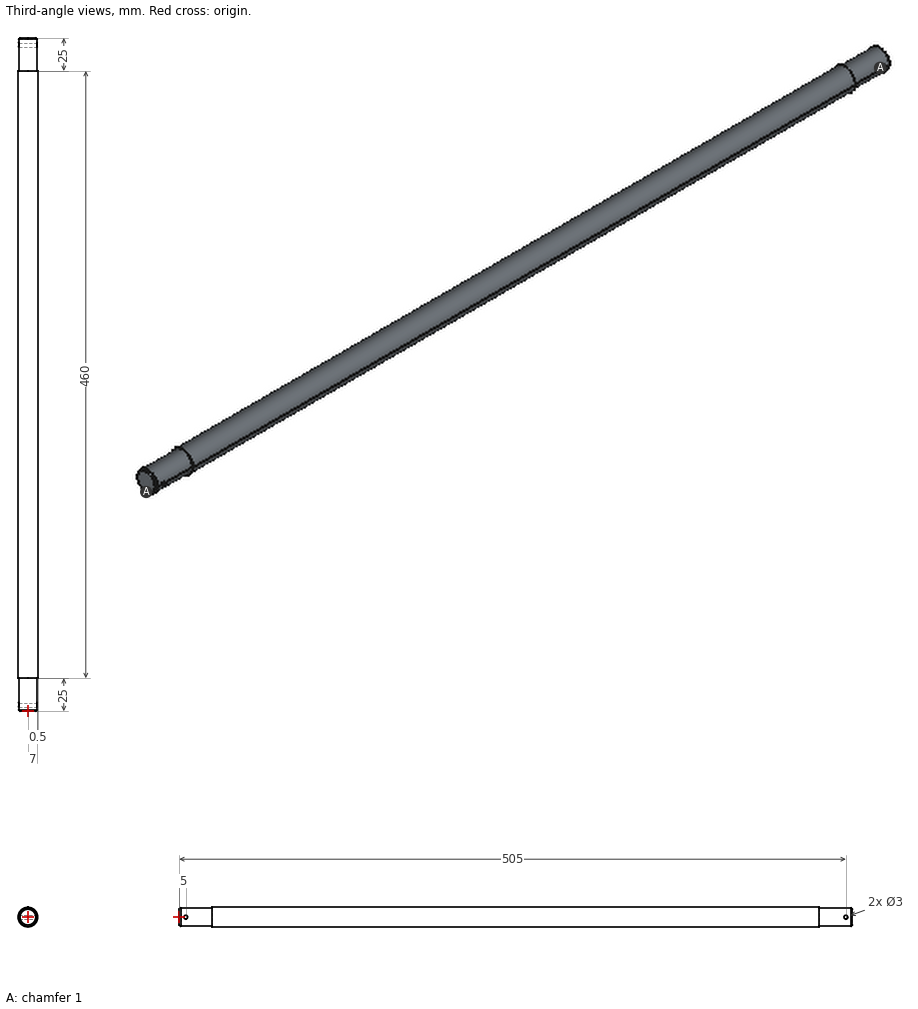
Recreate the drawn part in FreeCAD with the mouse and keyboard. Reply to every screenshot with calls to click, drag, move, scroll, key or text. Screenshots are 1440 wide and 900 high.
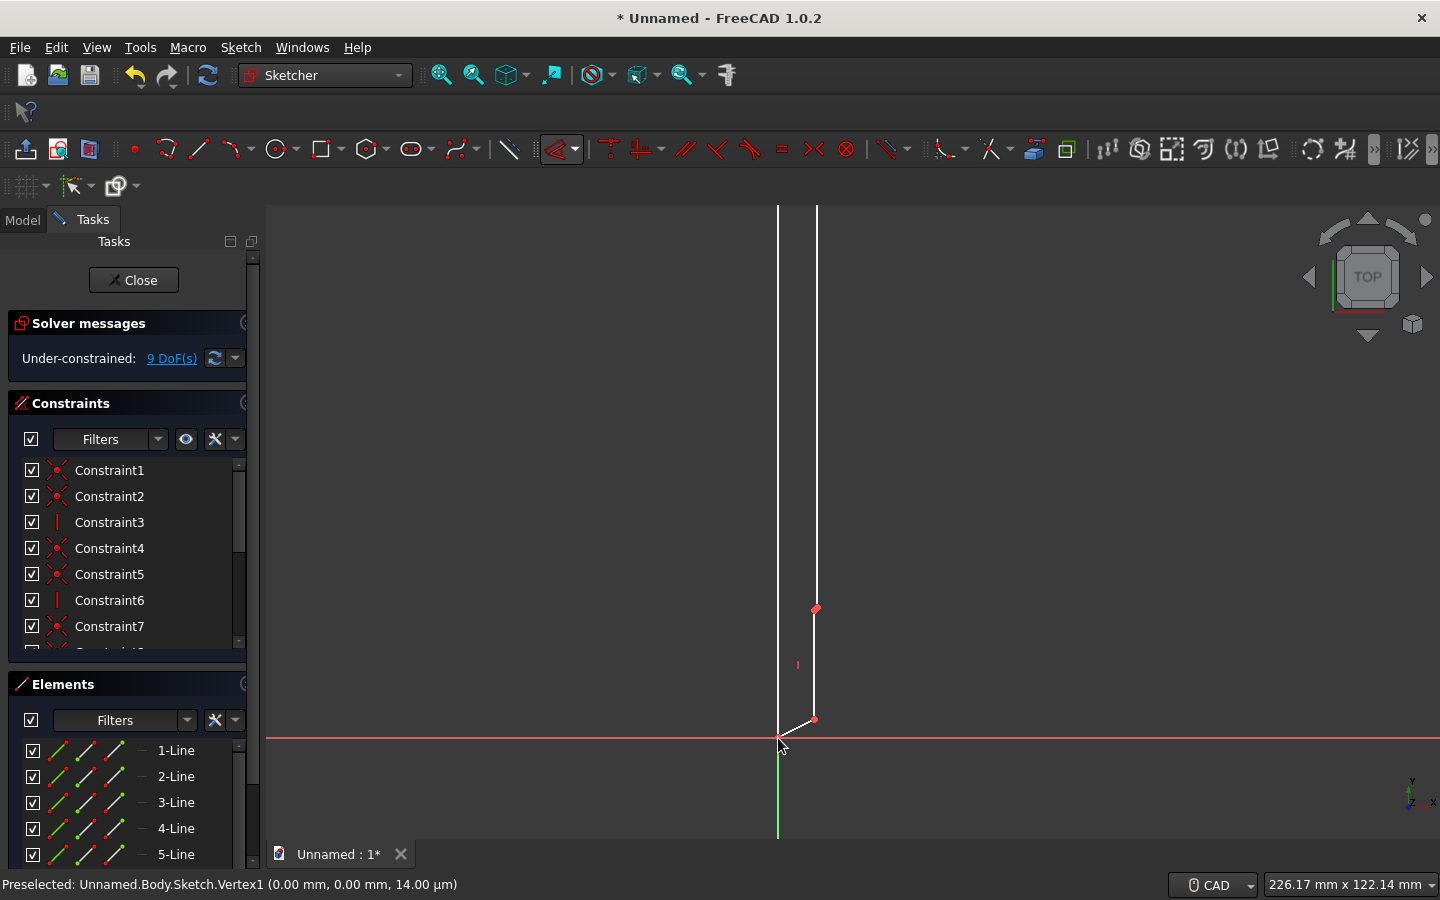
click(804, 725)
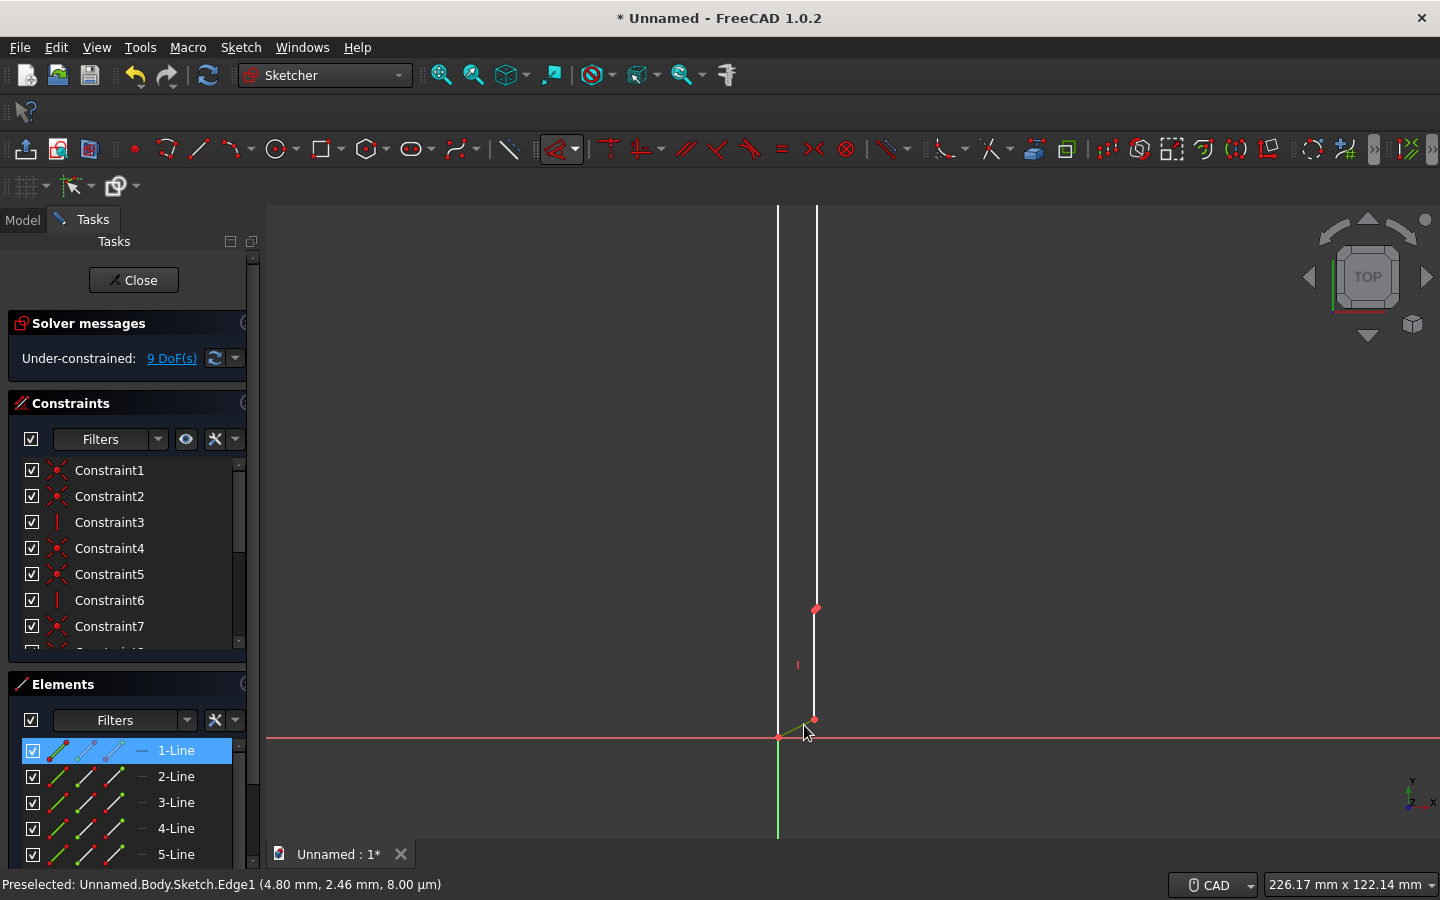
click(664, 150)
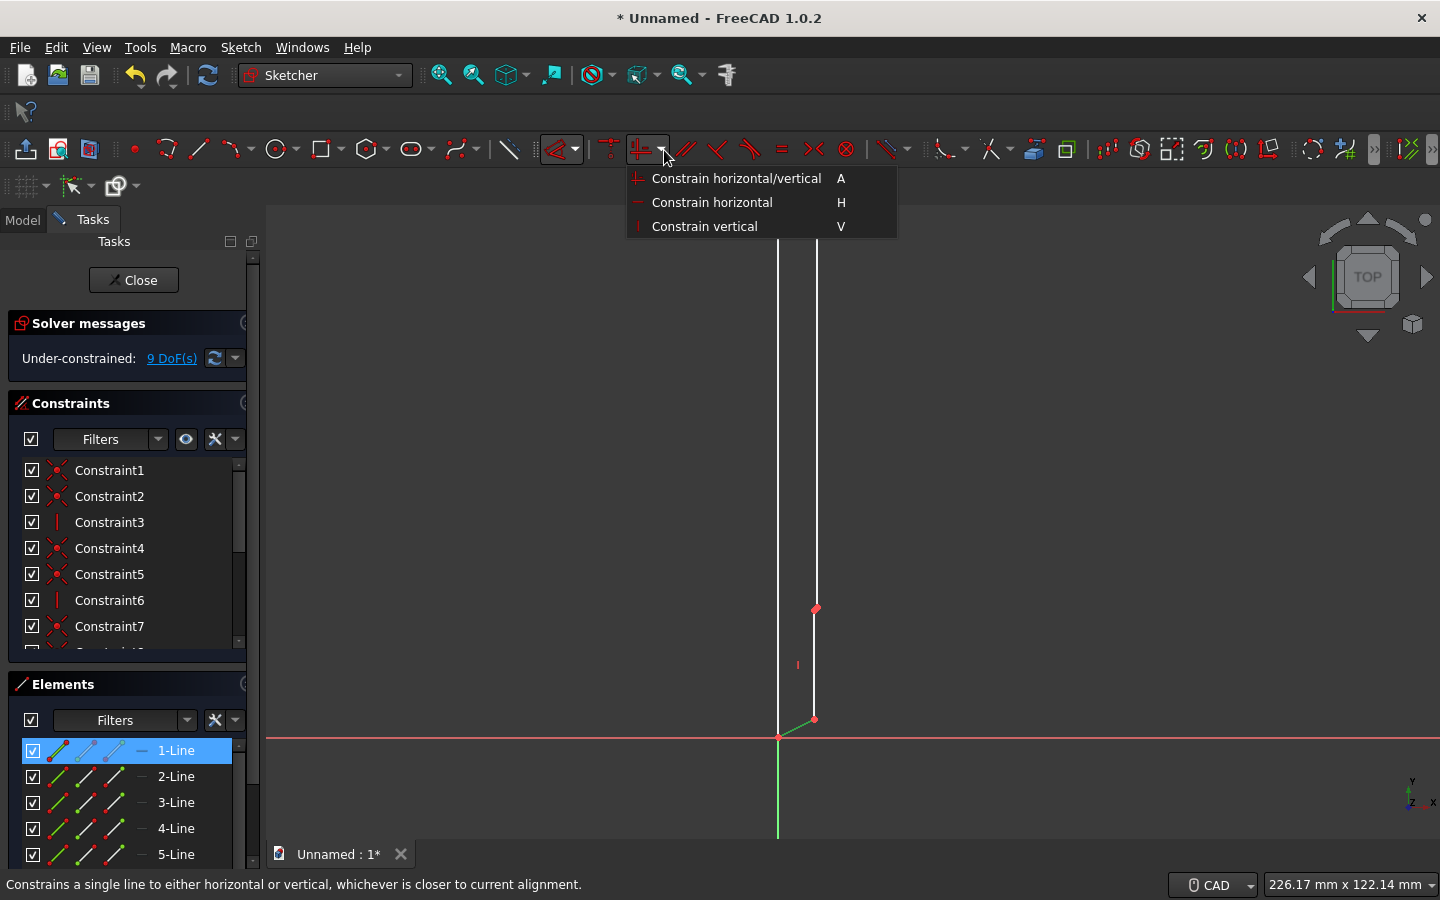
click(762, 202)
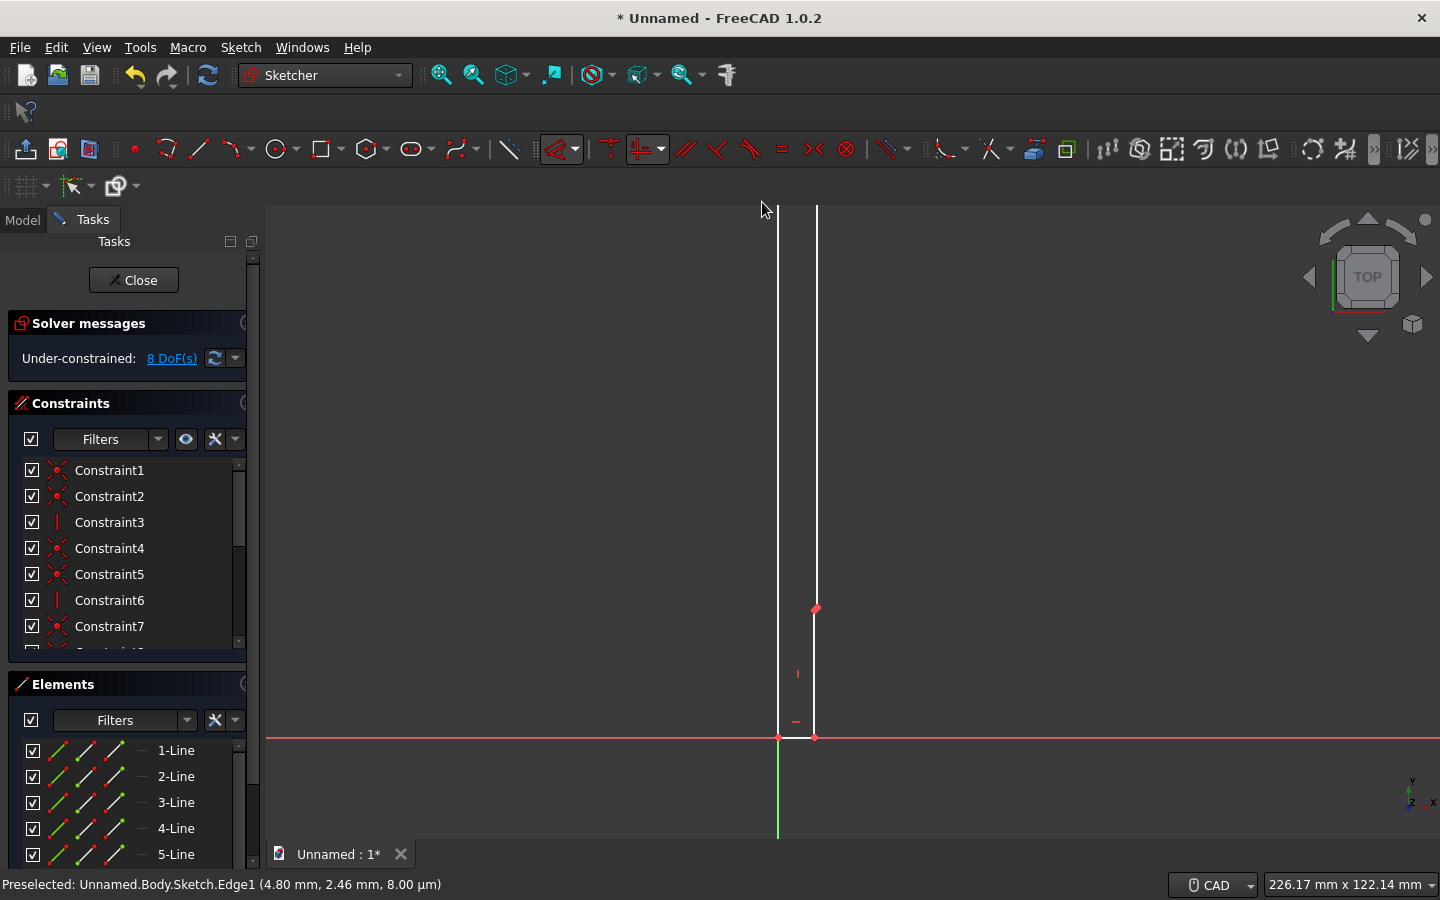
scroll(816, 609, up, 5)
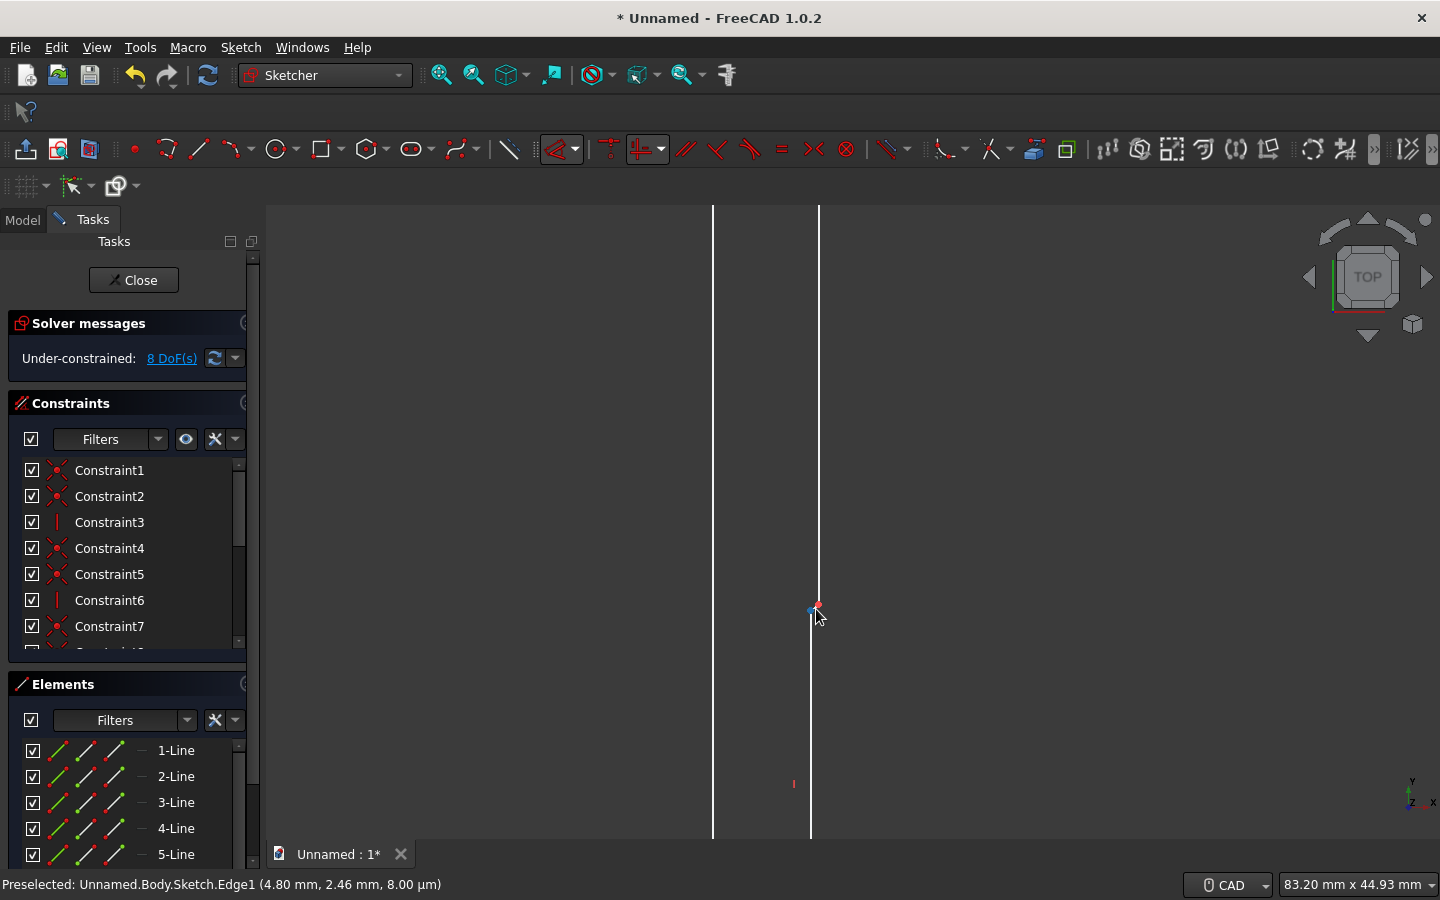
scroll(815, 608, up, 4)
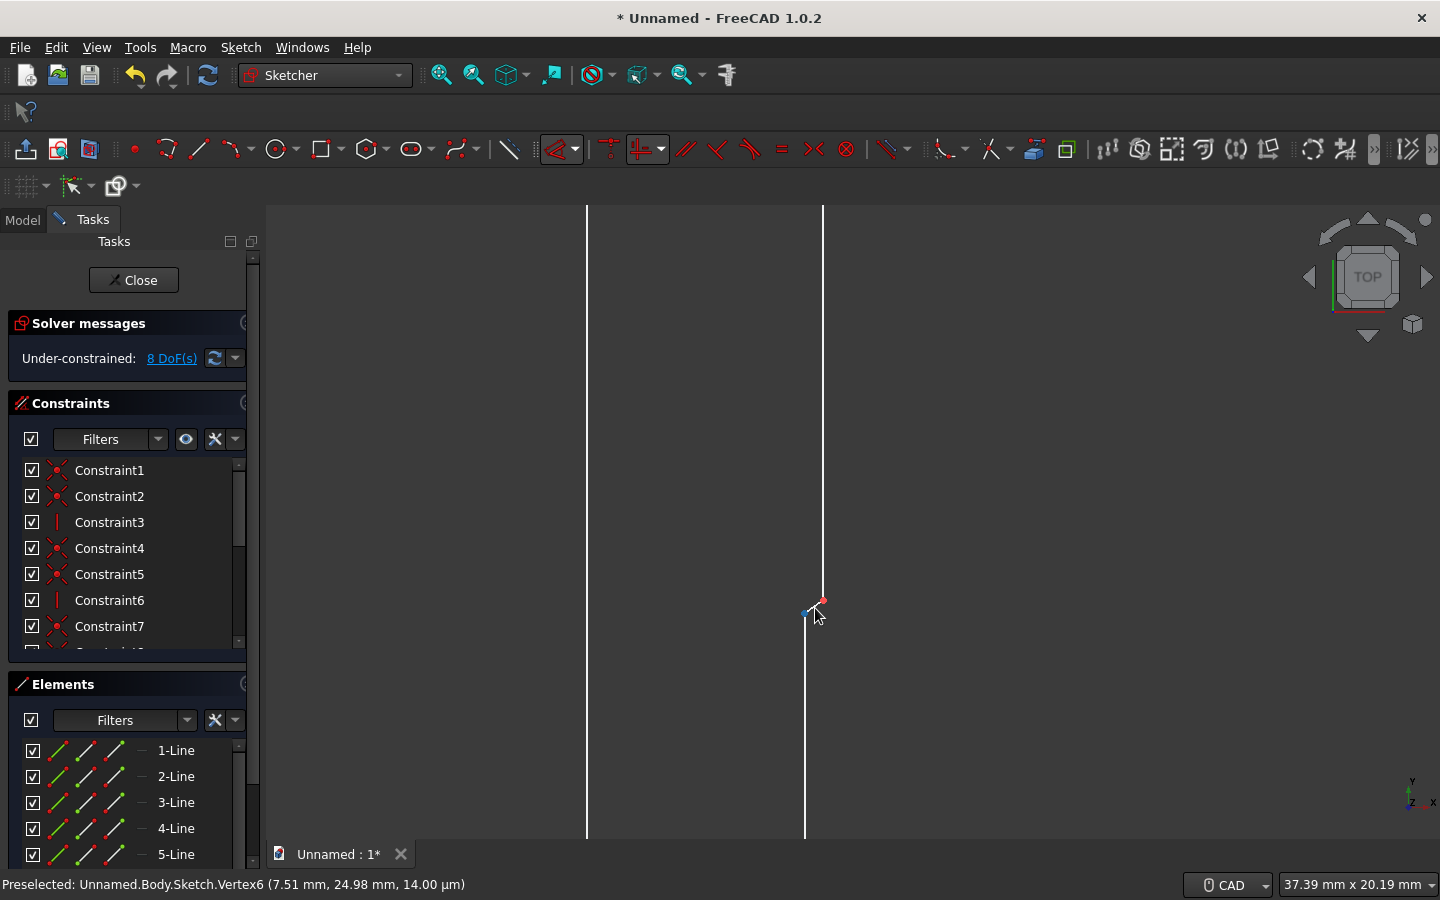
click(814, 607)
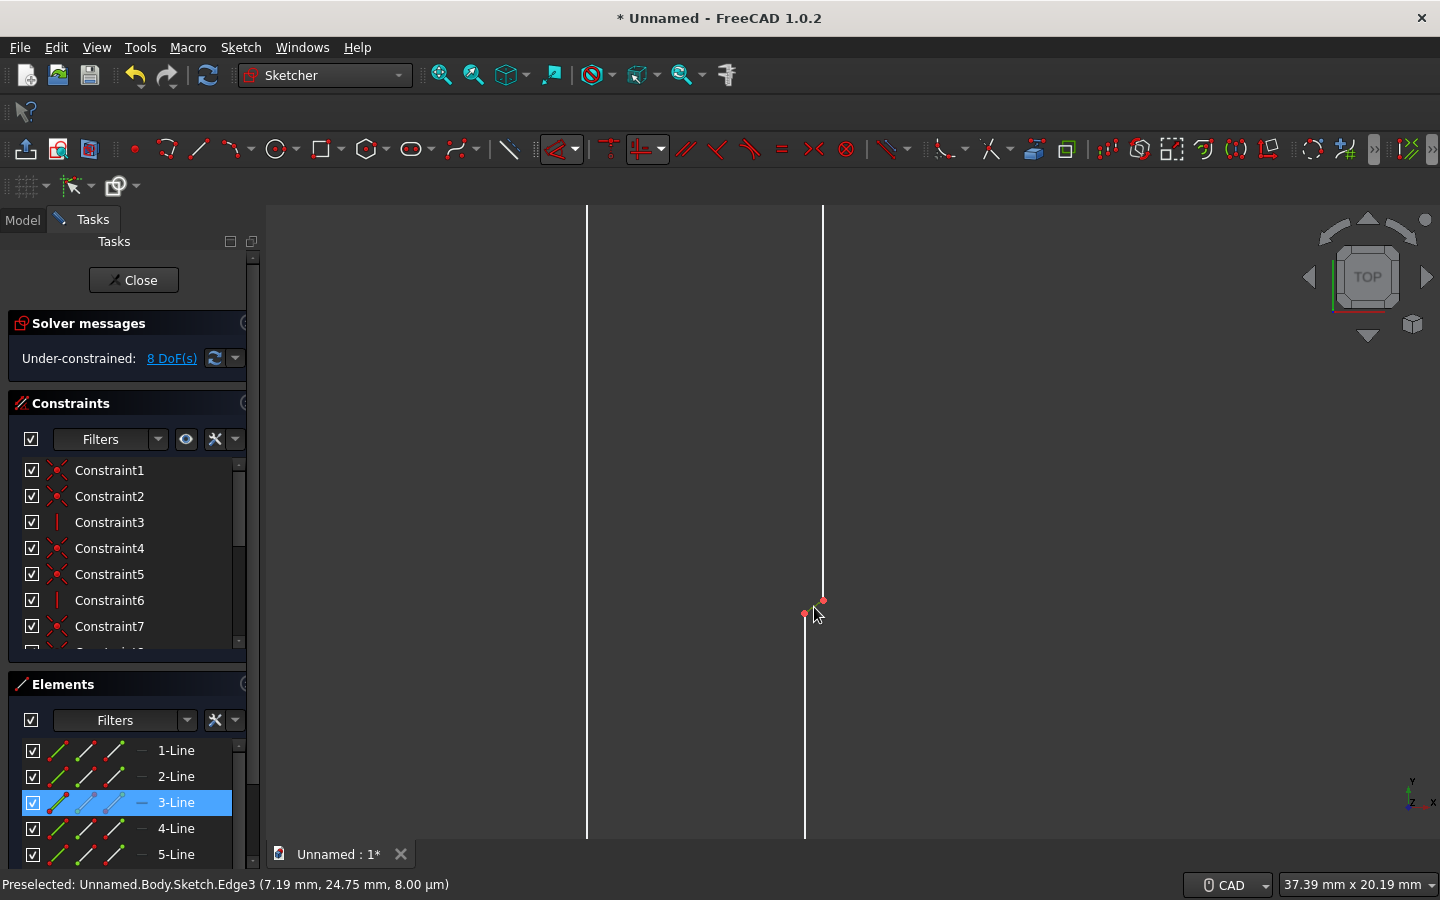
click(664, 150)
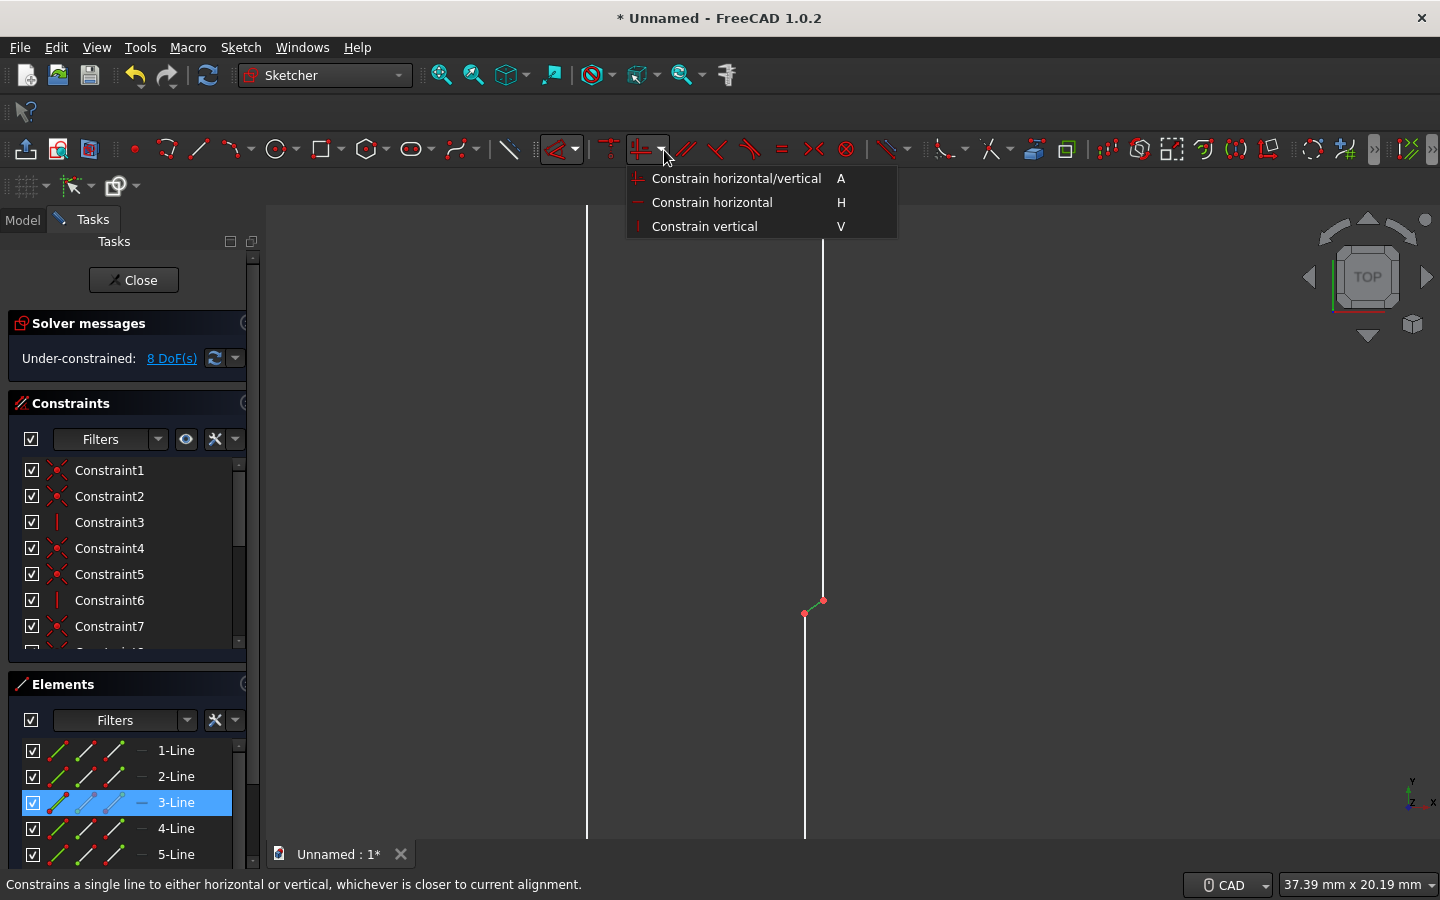
click(762, 202)